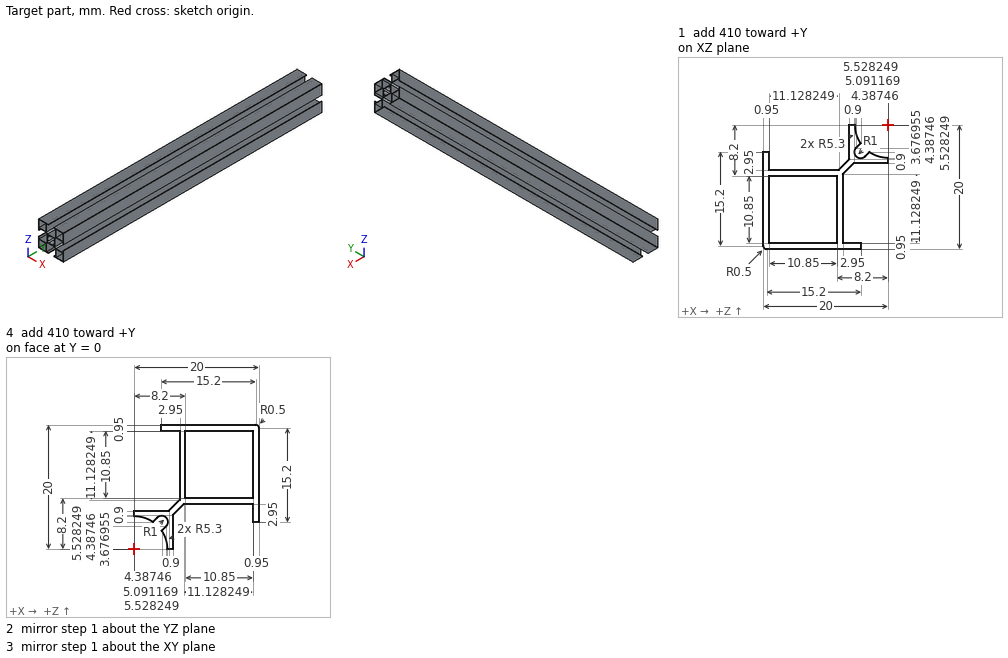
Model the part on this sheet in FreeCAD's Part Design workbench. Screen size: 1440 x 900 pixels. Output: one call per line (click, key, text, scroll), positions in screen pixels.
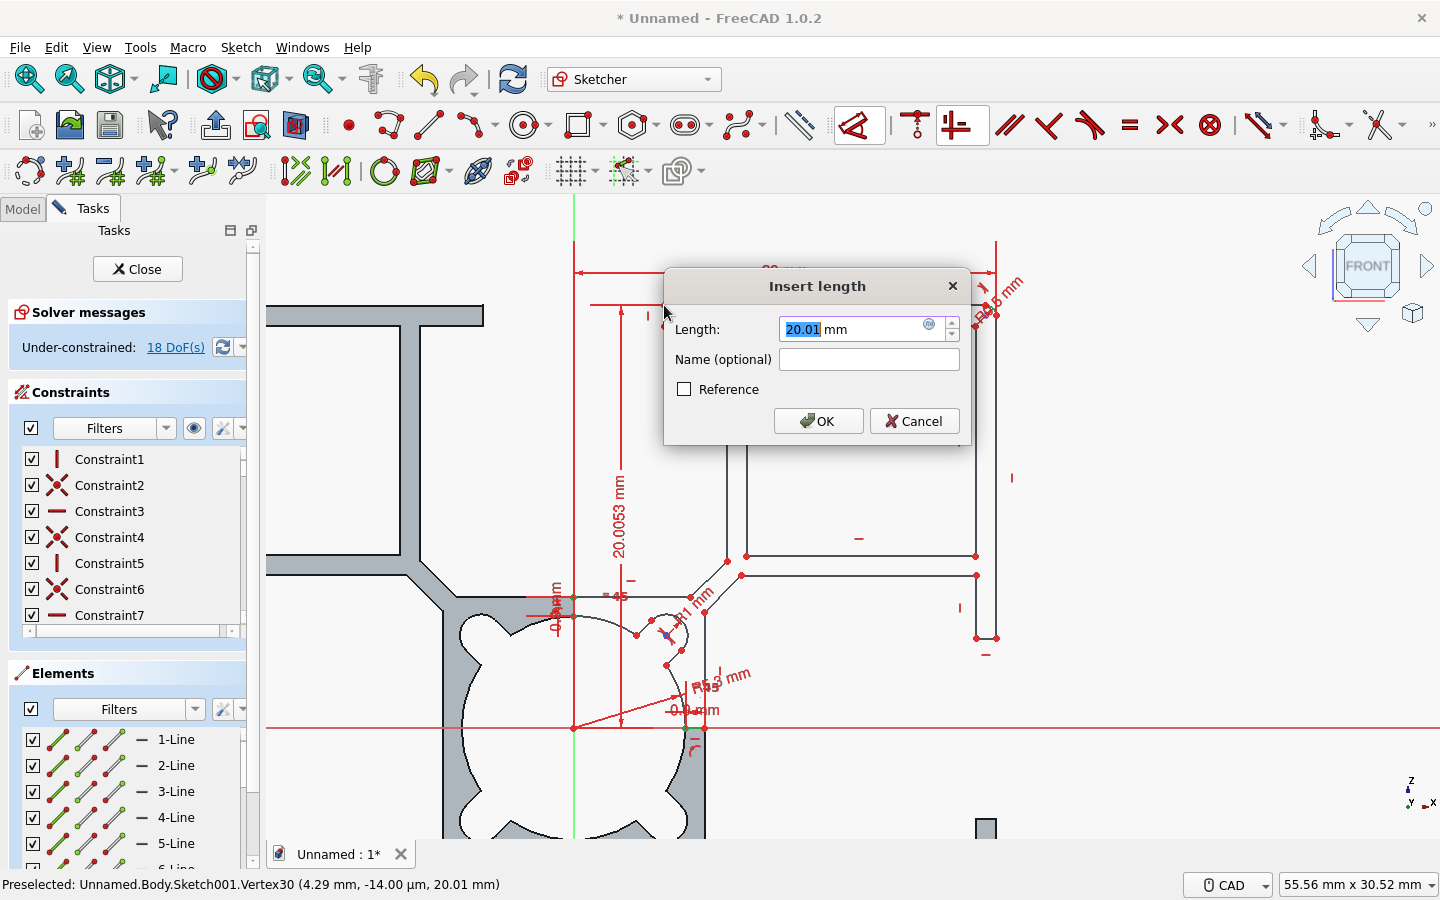
text(20)
key(Return)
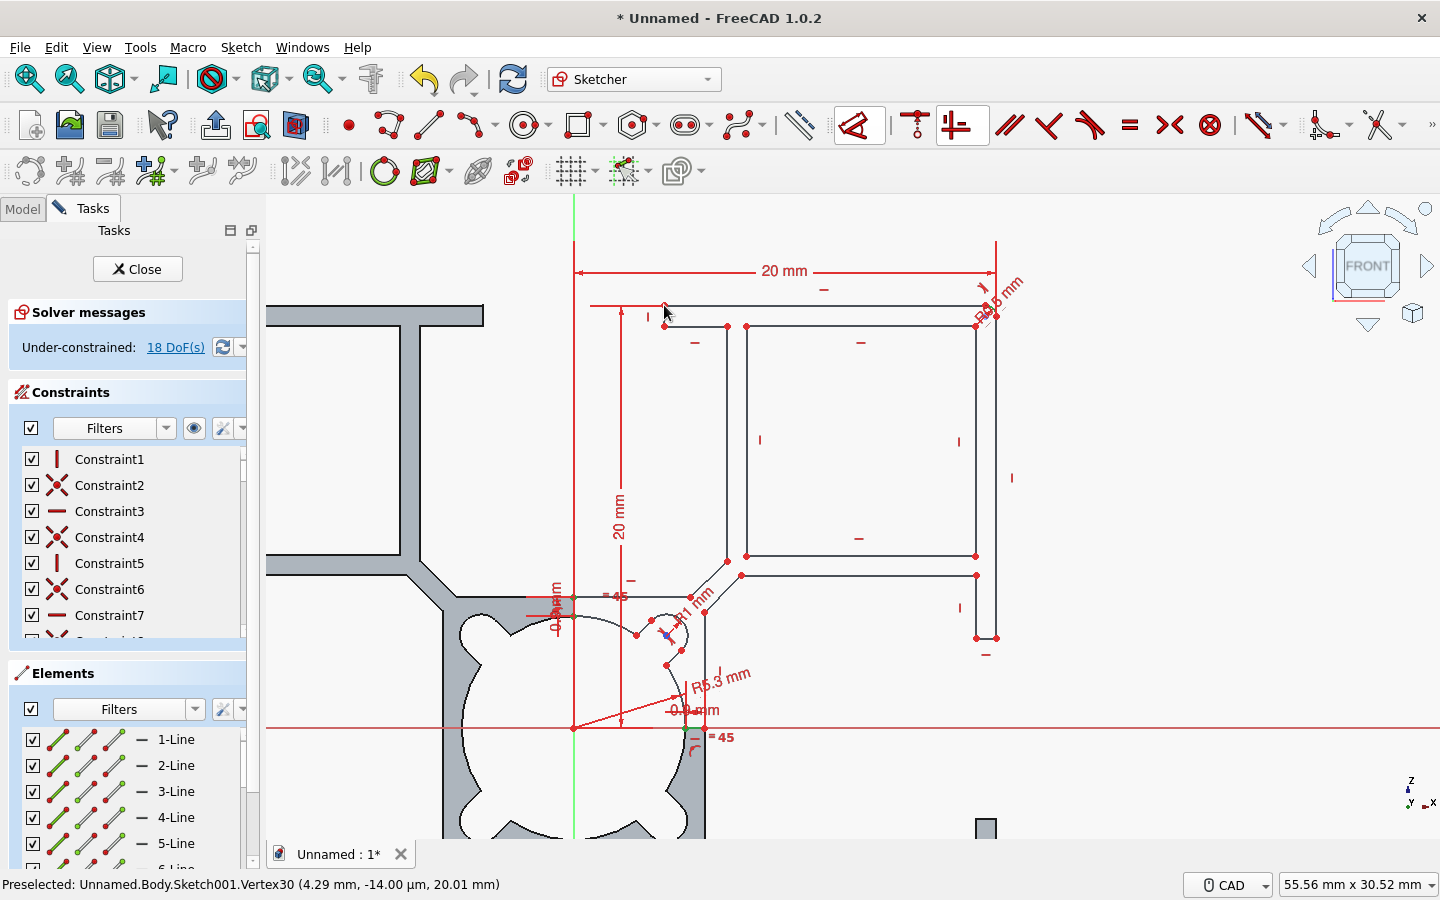
click(996, 413)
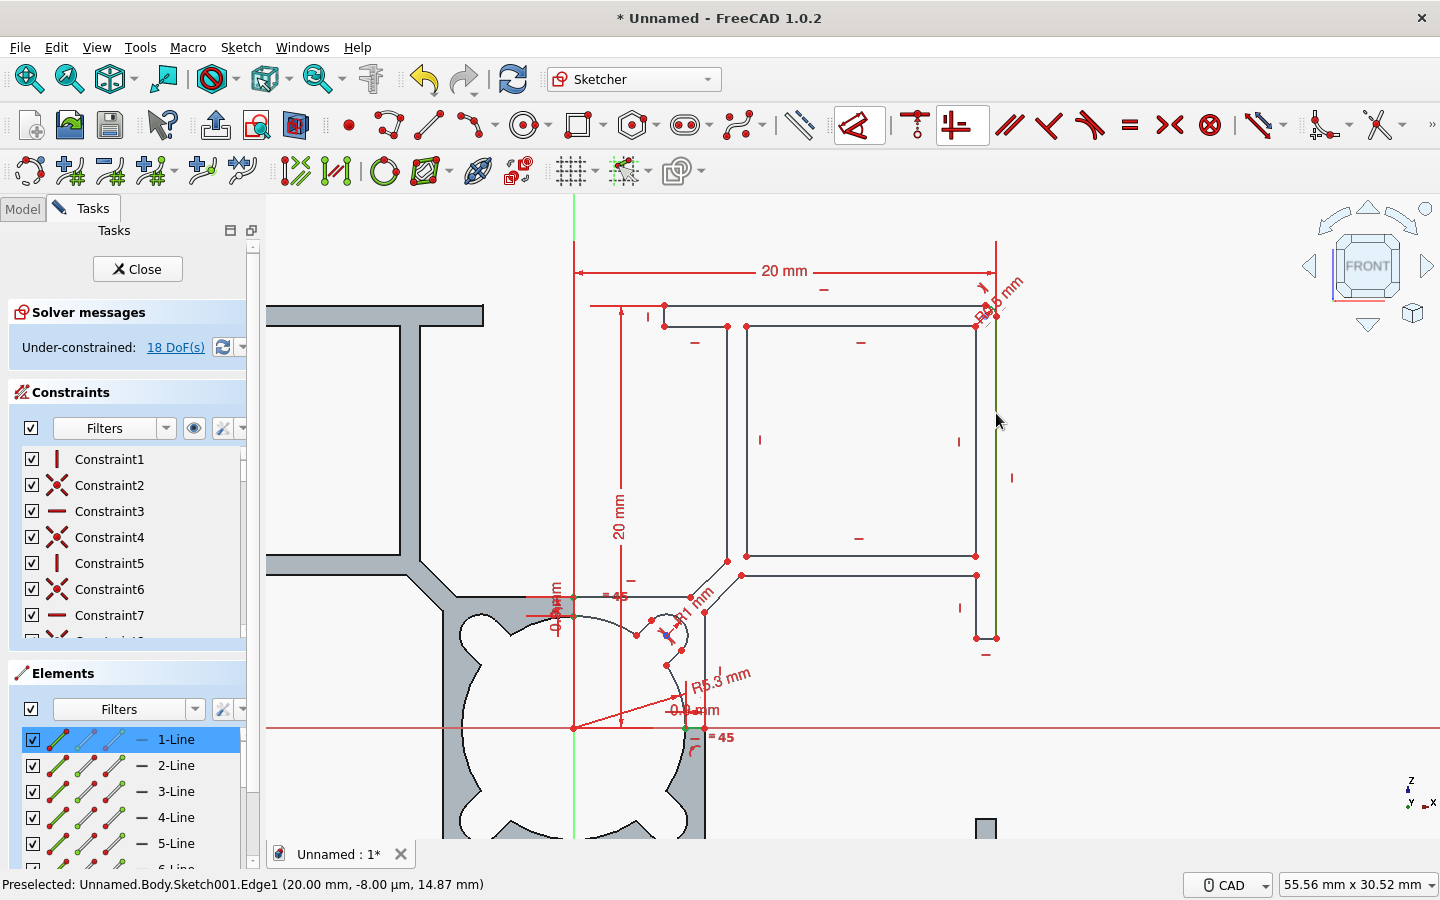
click(880, 126)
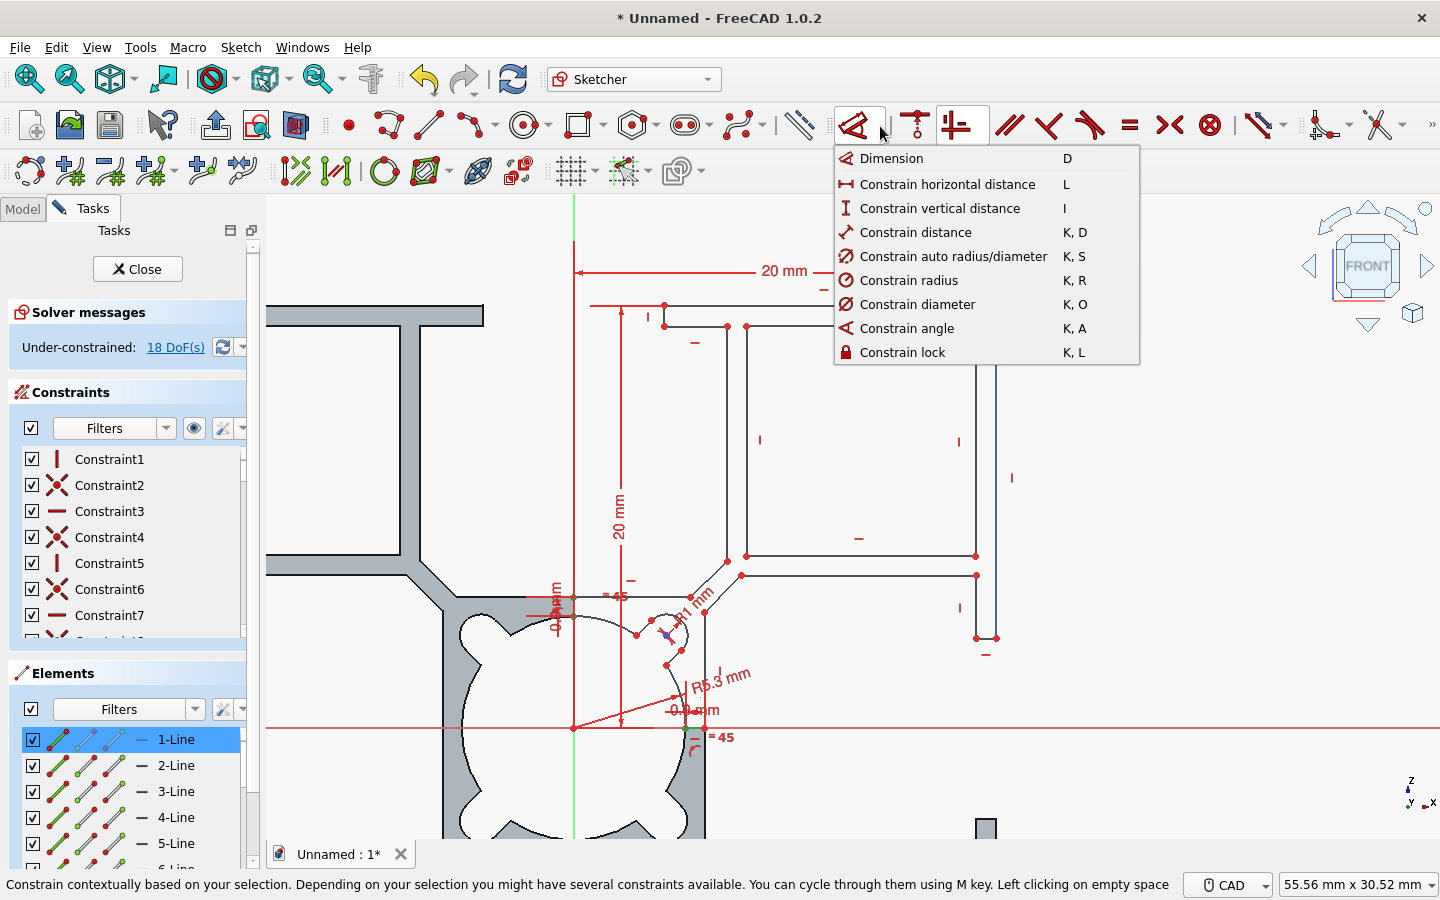
click(987, 208)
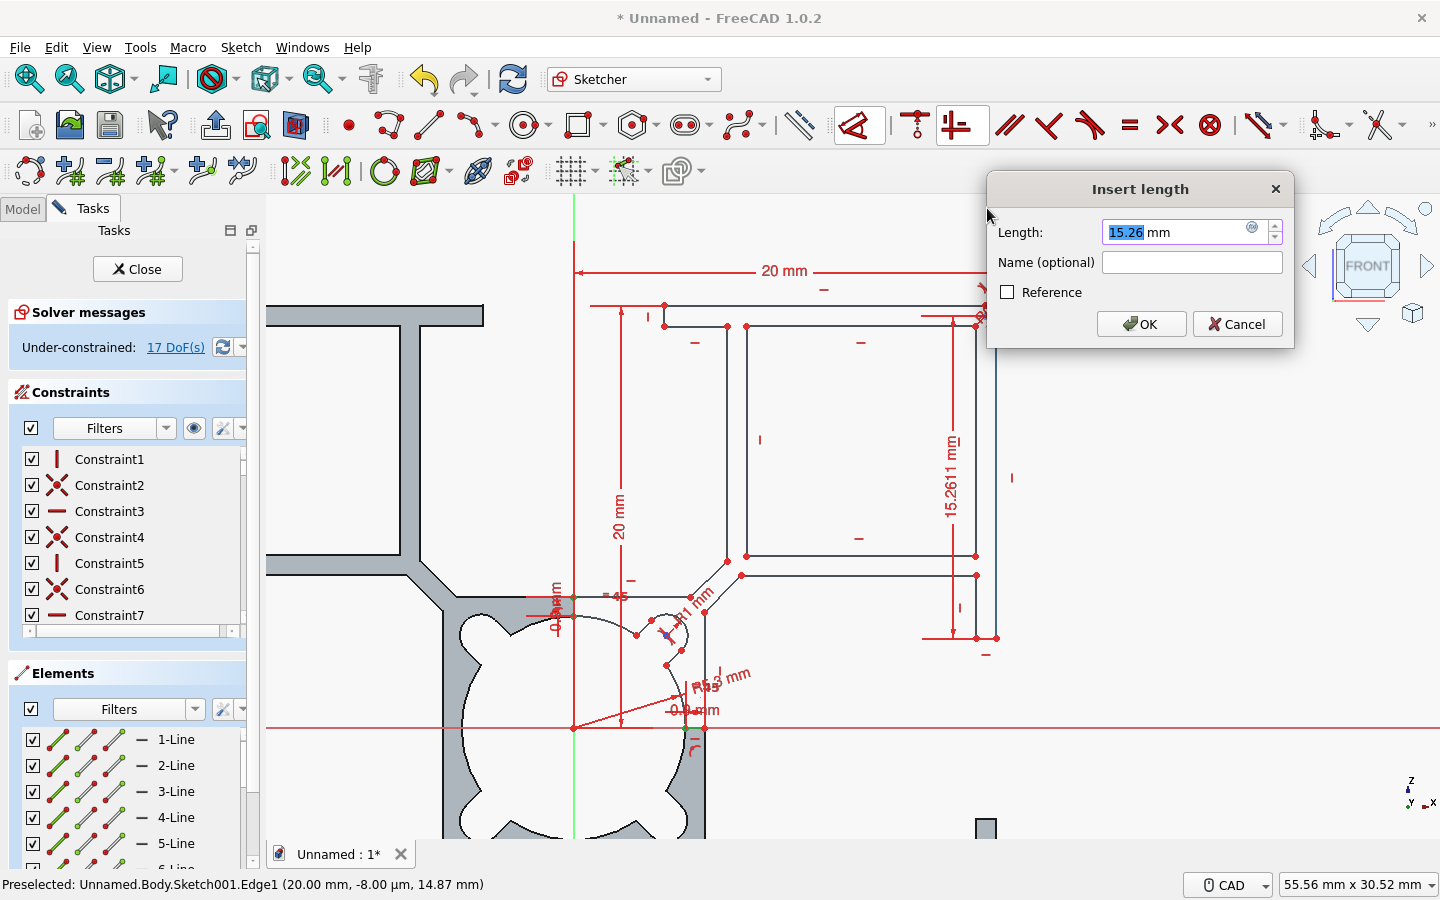
text(15.2)
key(Return)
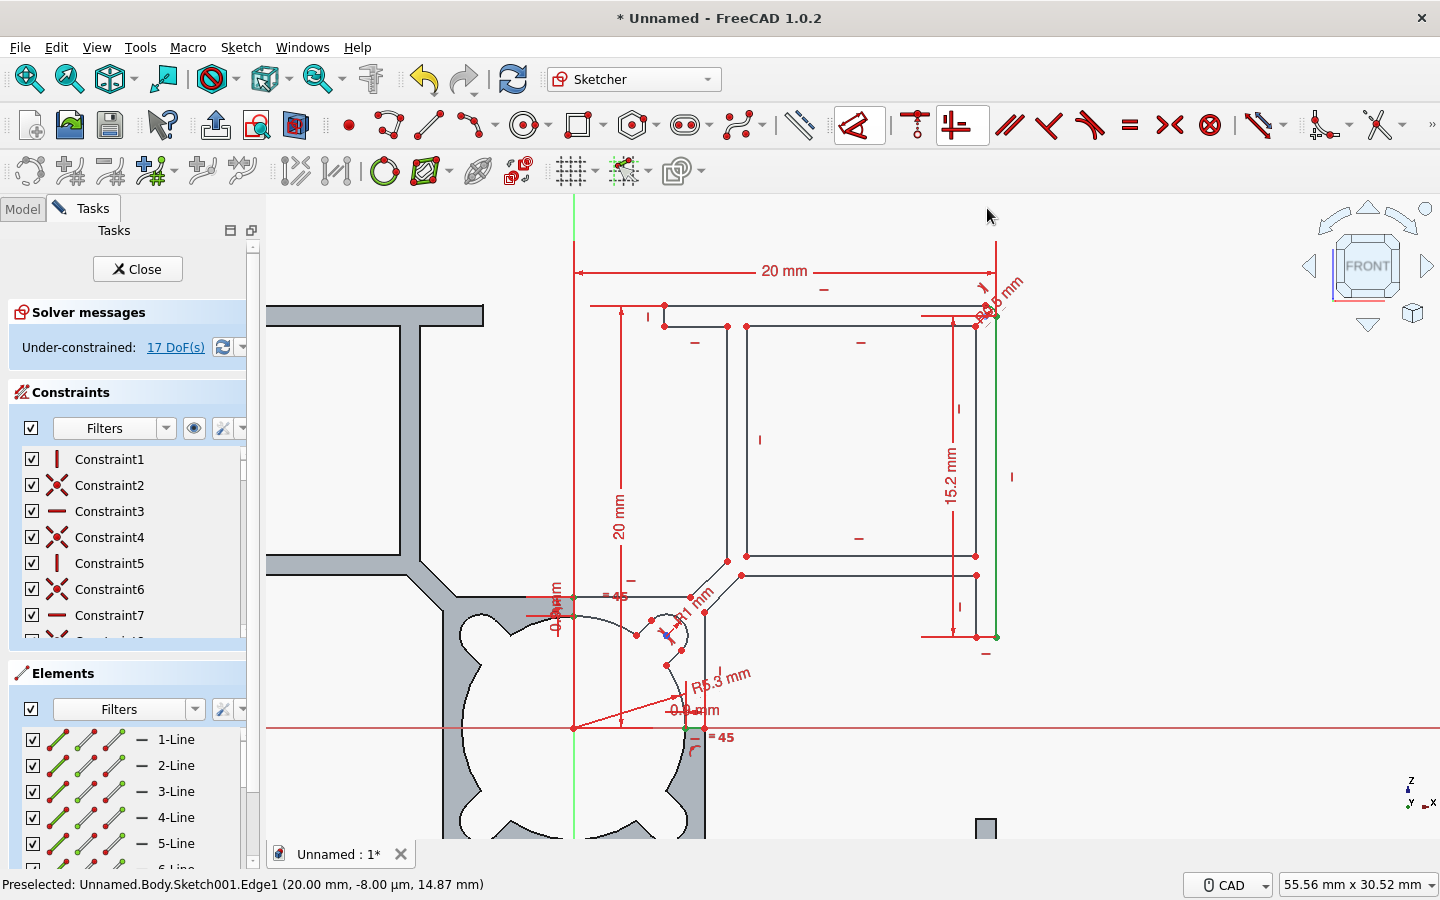
scroll(986, 637, up, 4)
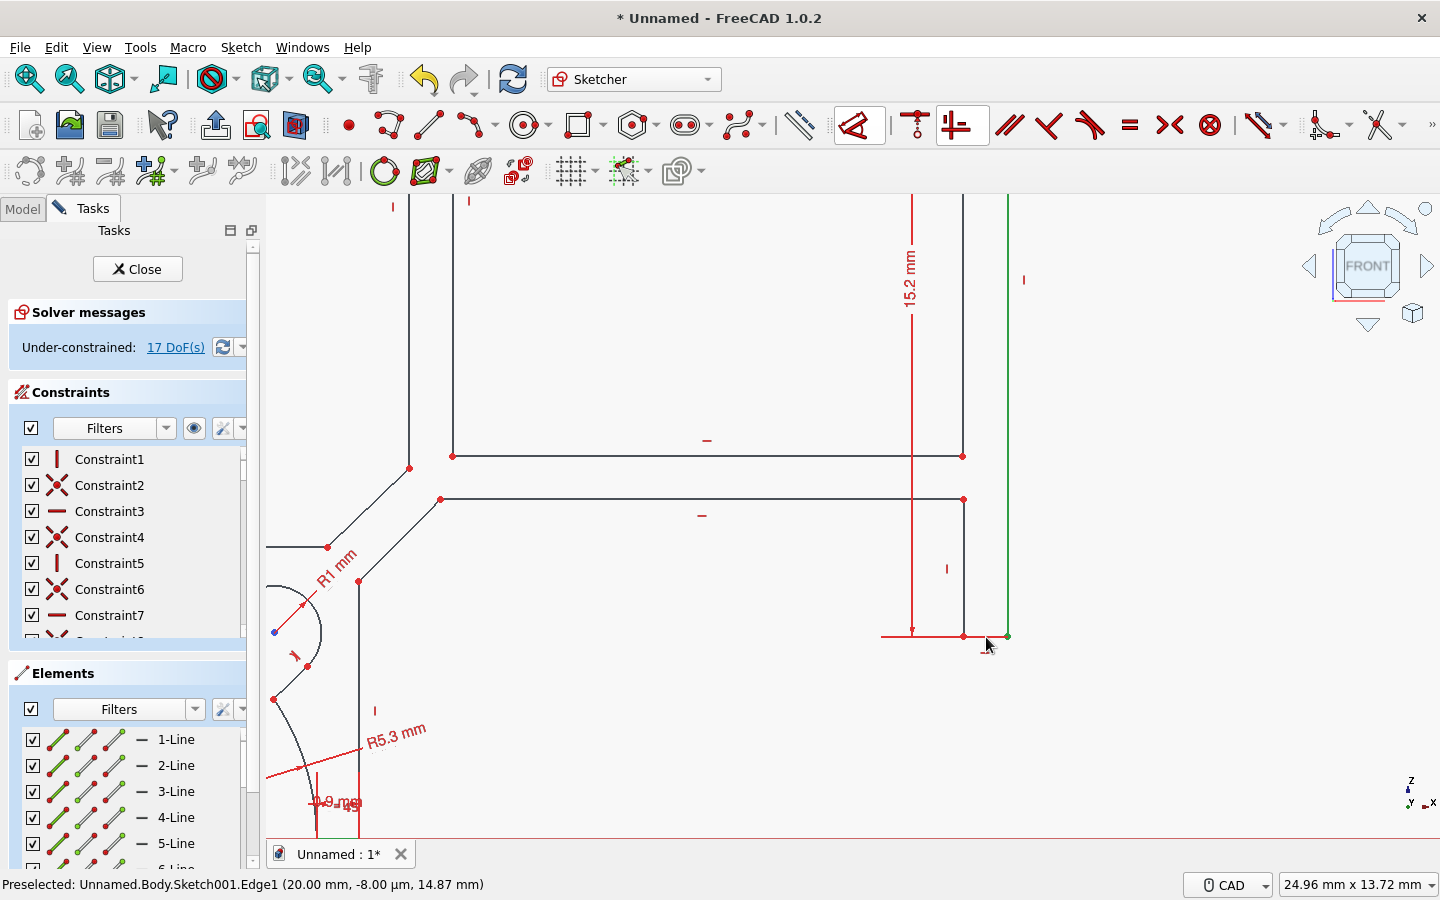
click(986, 637)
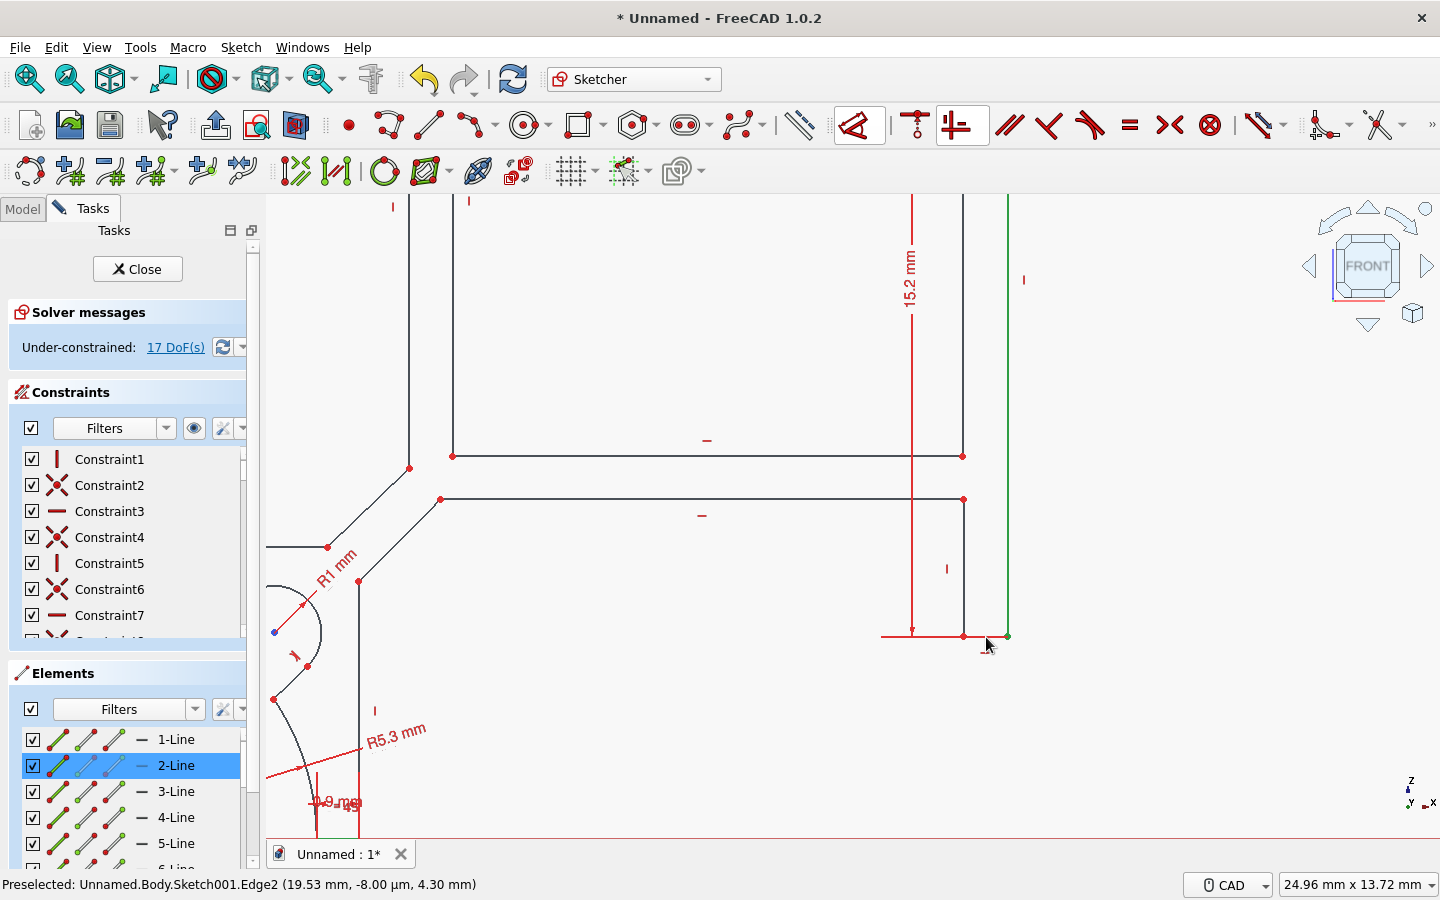
click(880, 126)